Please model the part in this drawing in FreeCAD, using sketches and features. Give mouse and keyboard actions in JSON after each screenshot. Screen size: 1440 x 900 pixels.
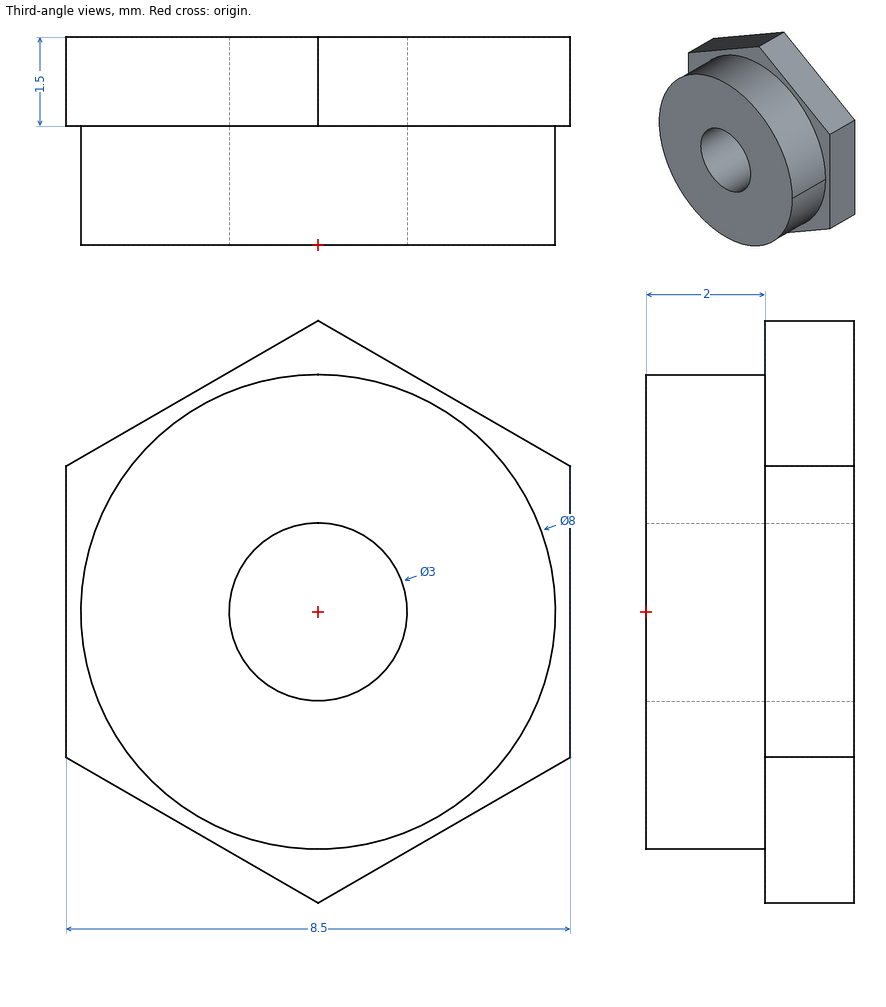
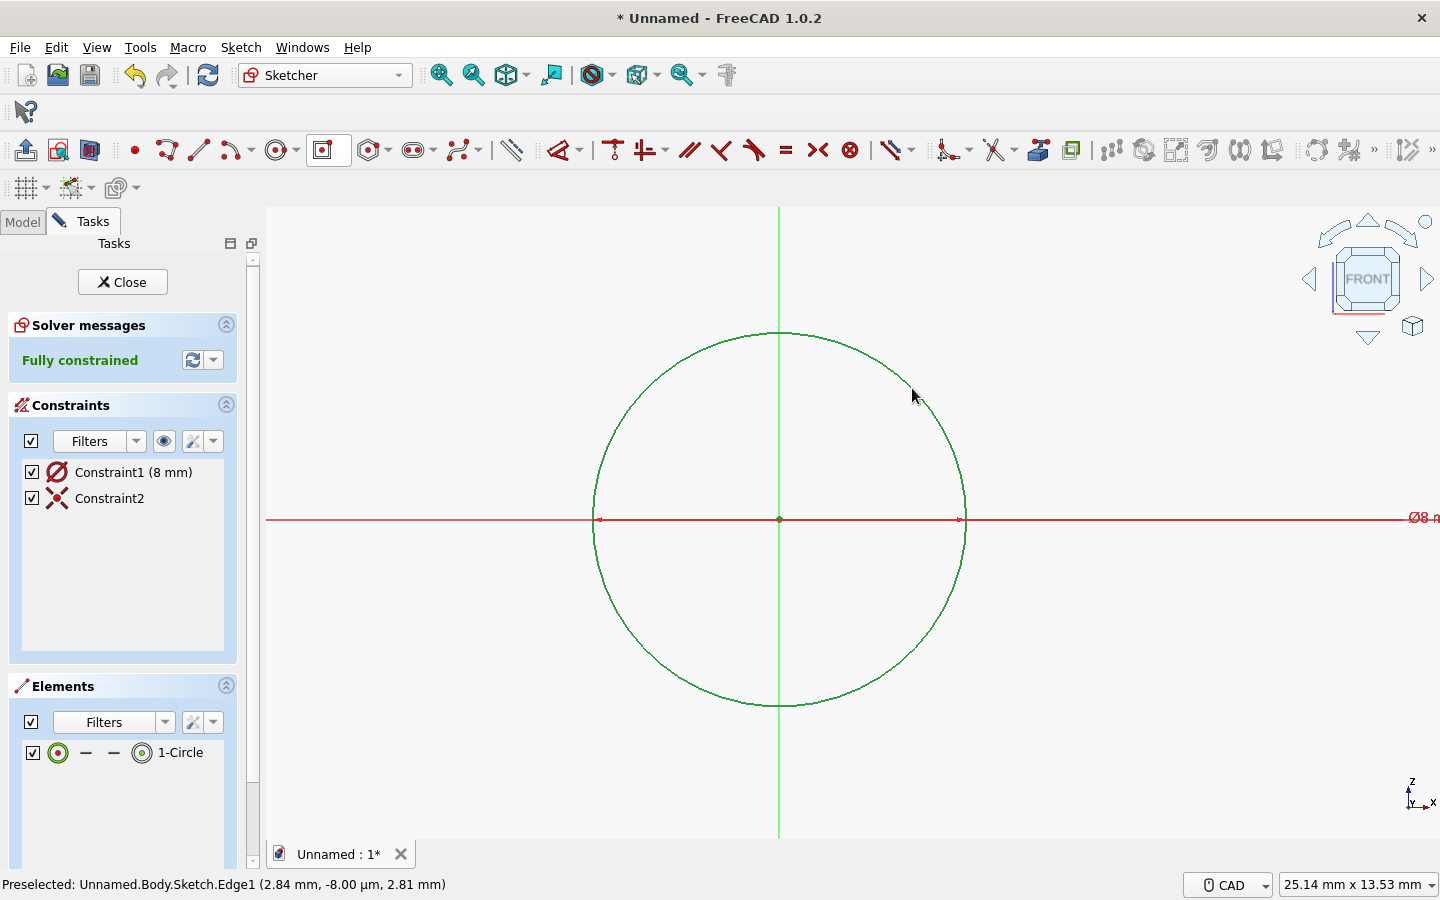
{"action": "left_click", "coordinate": [123, 282]}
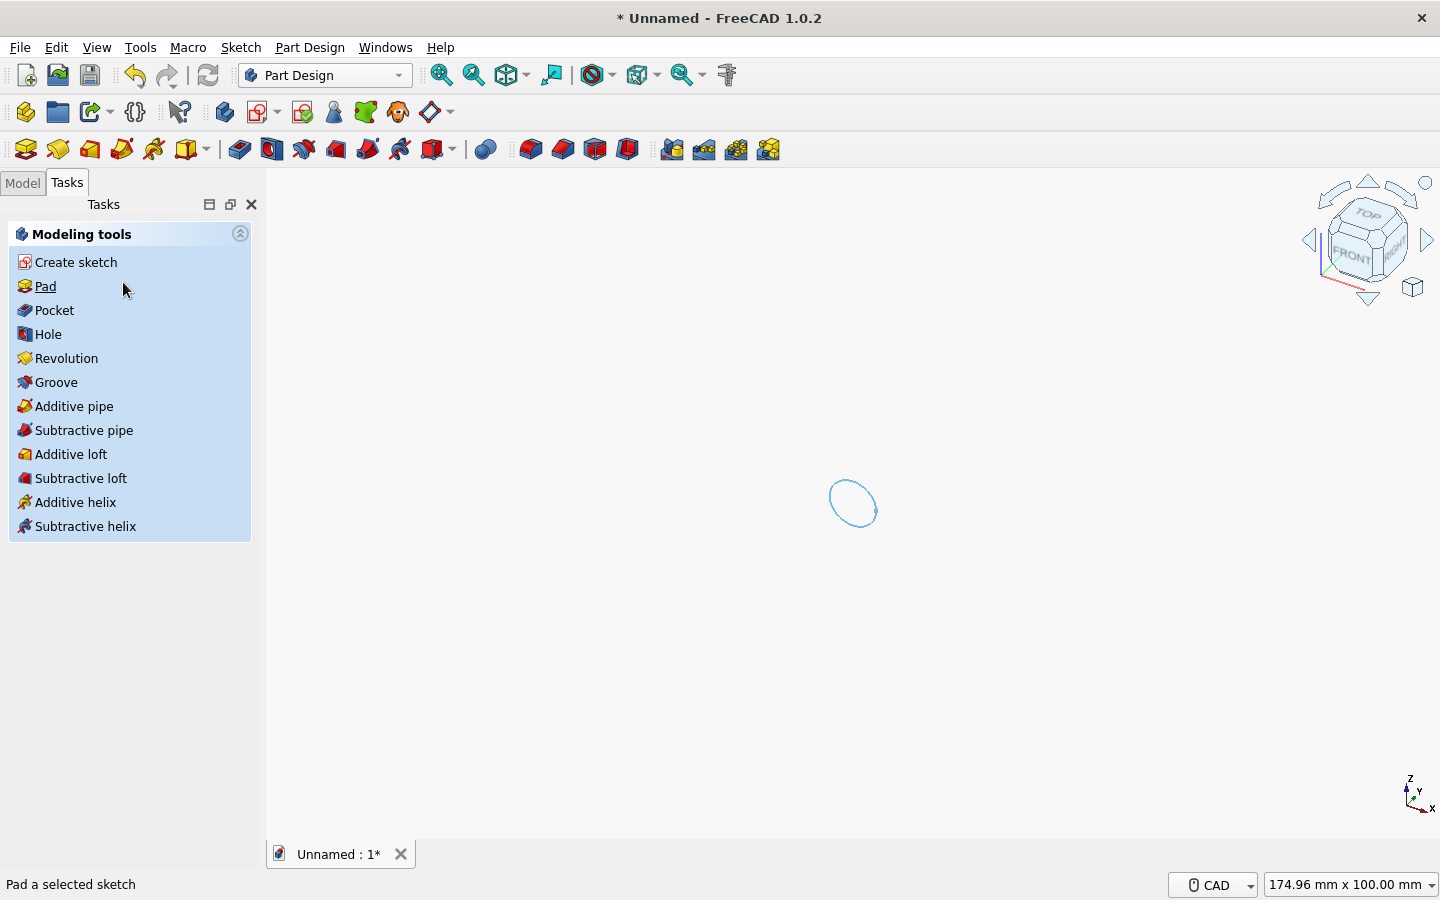
{"action": "left_click", "coordinate": [26, 150]}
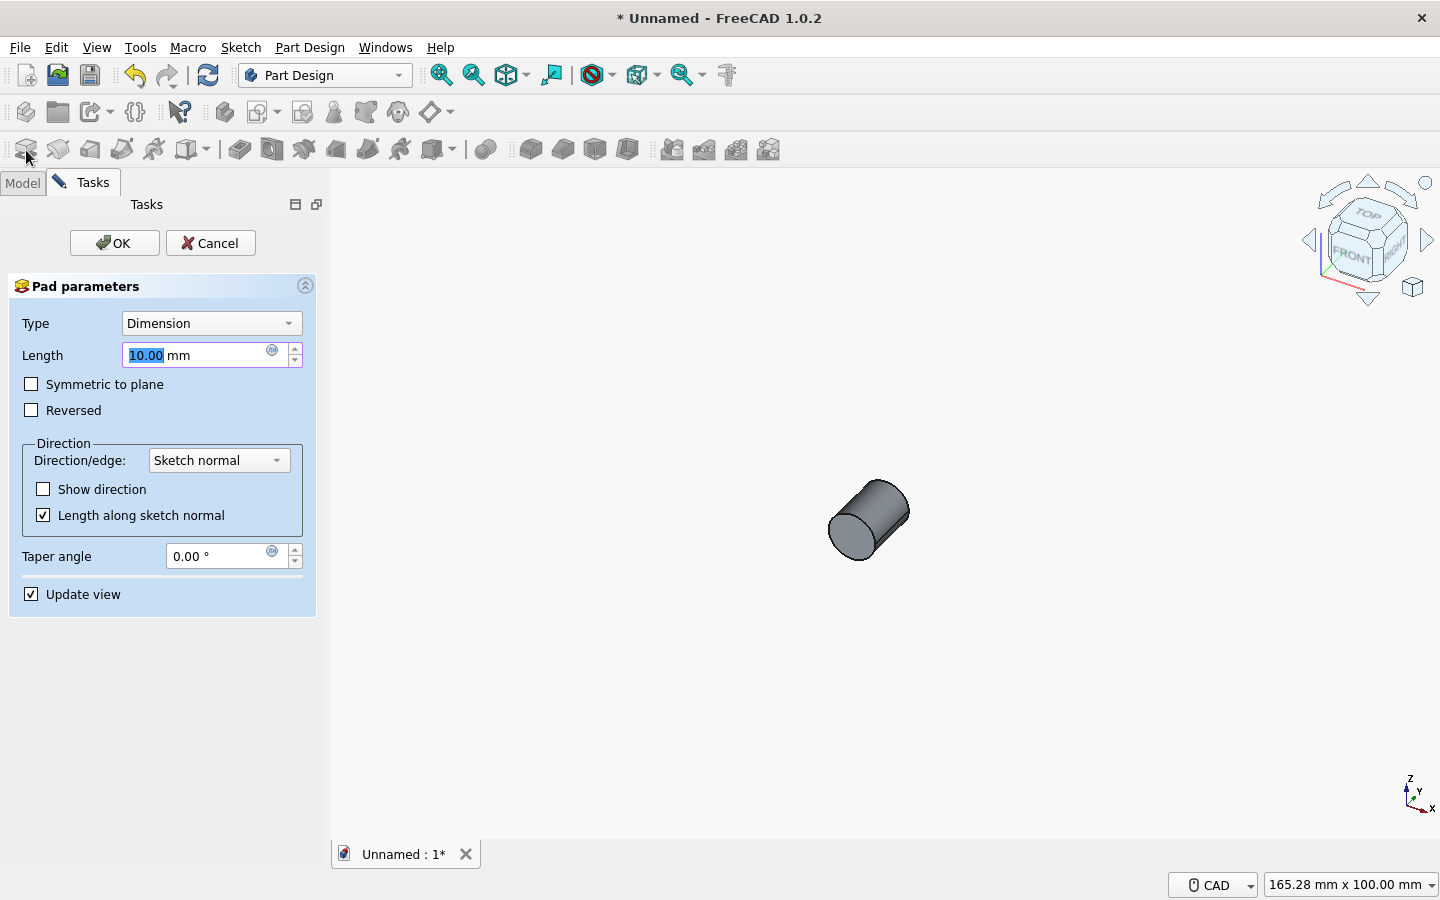
{"action": "type", "text": "2"}
{"action": "key", "text": "Tab"}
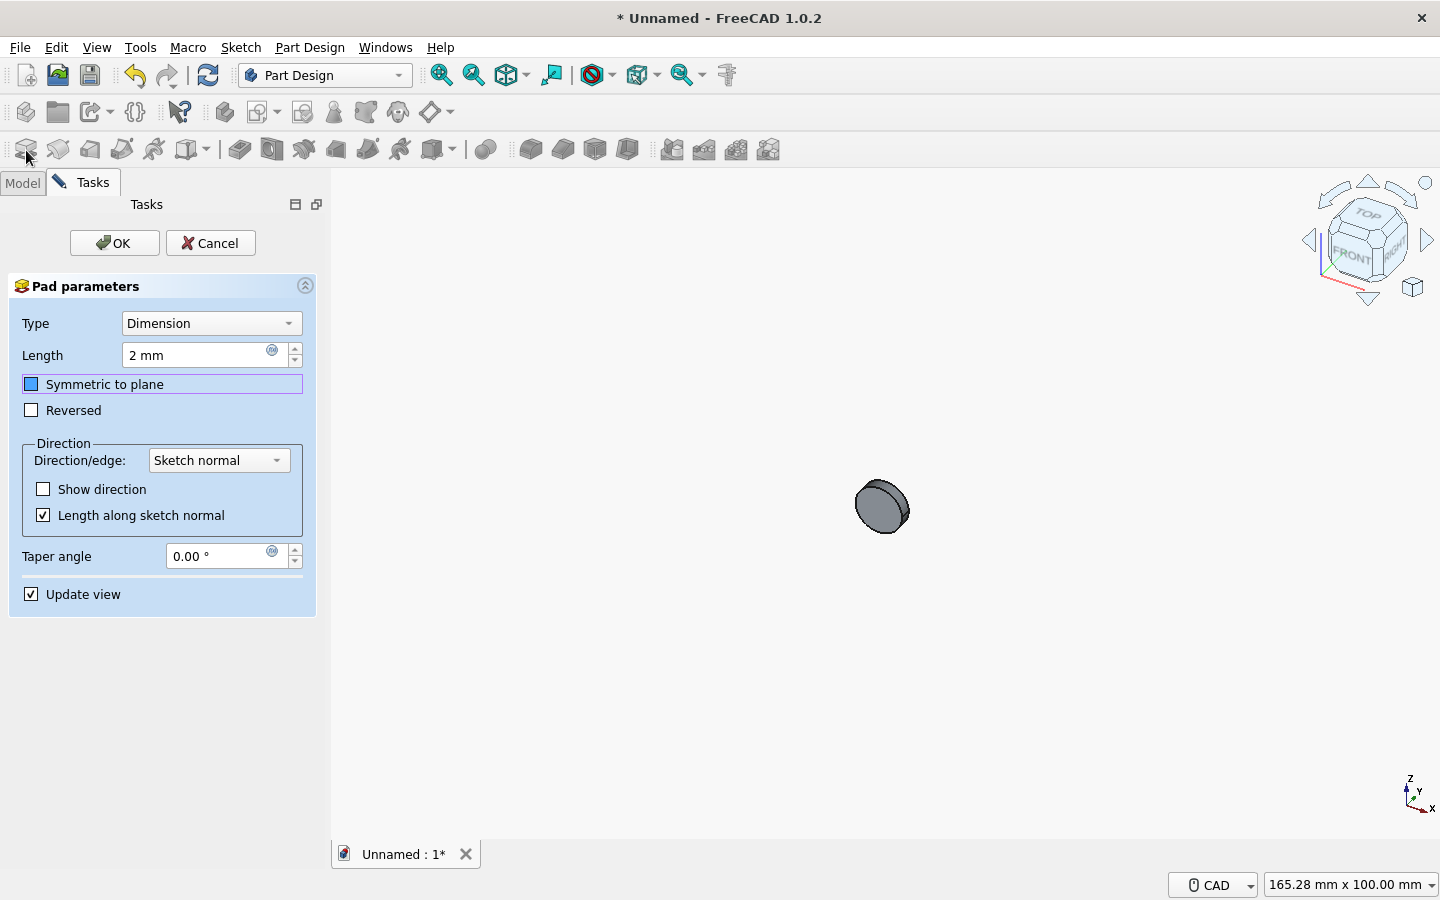
{"action": "left_click", "coordinate": [30, 410]}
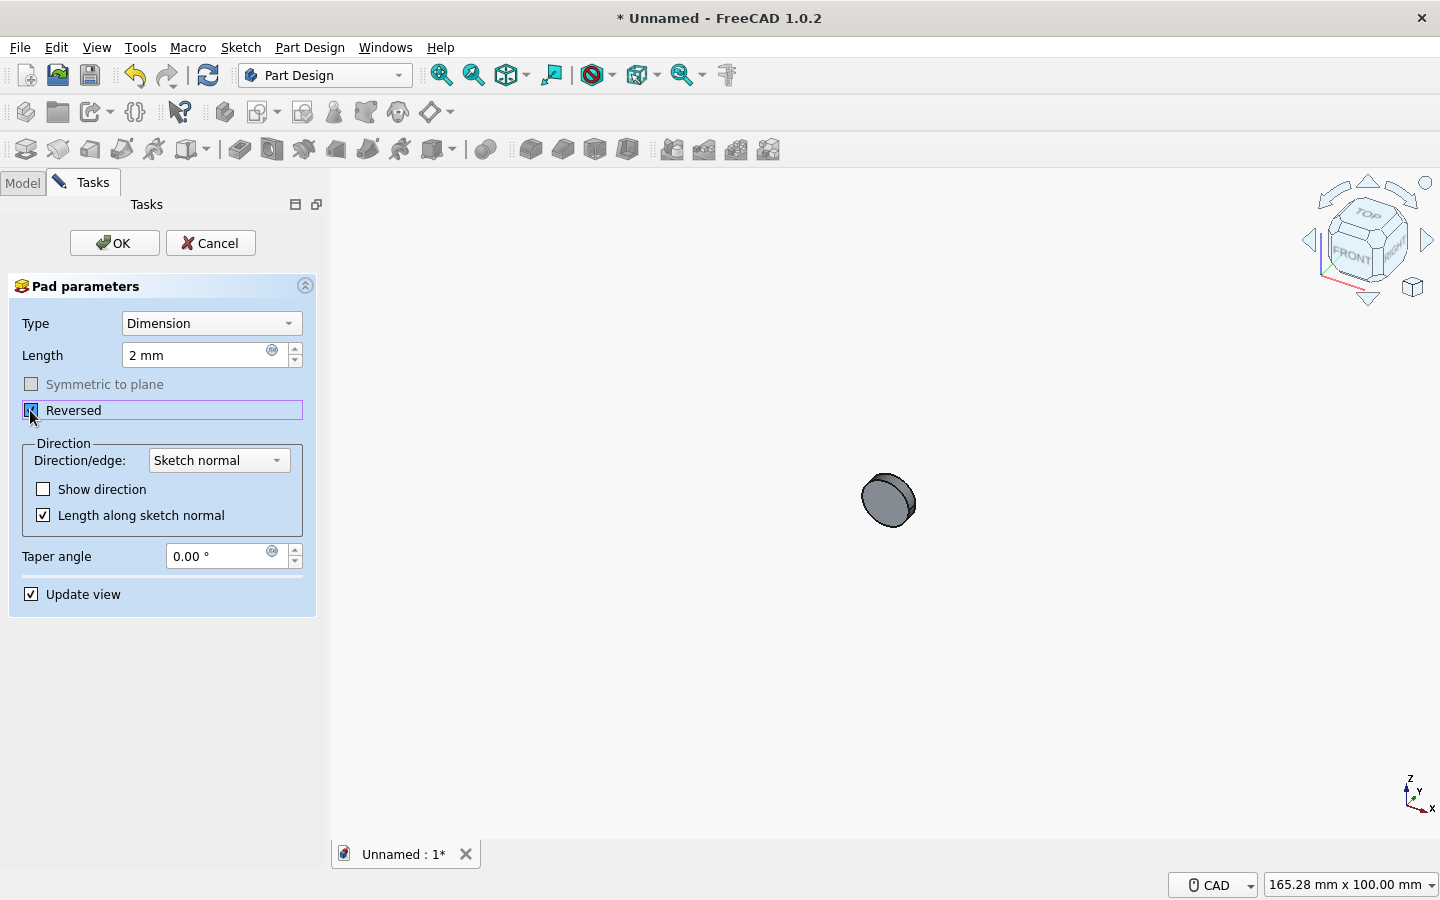
{"action": "left_click", "coordinate": [115, 243]}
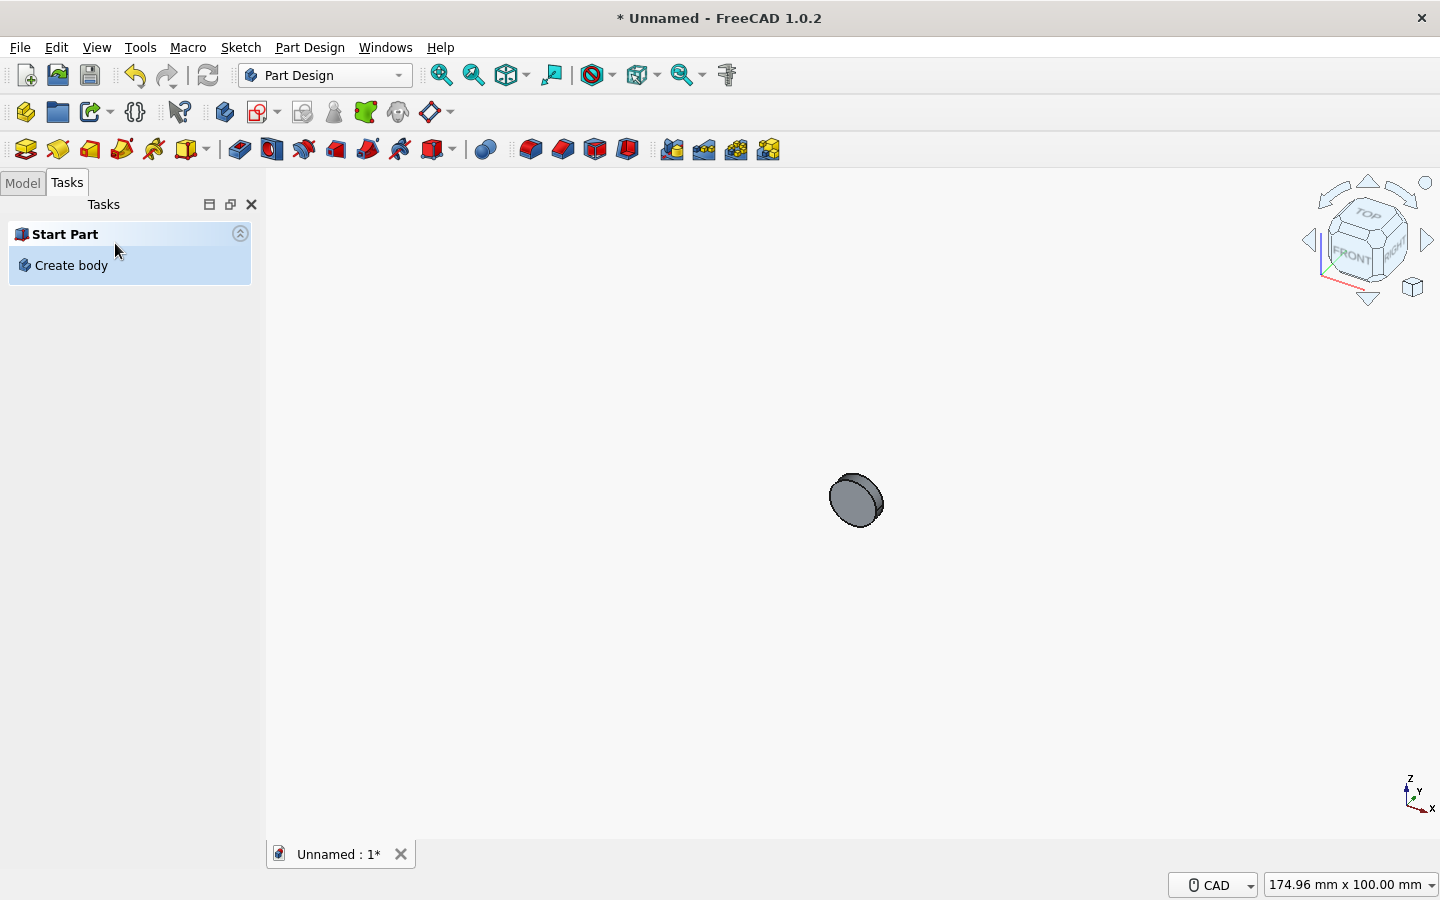
{"action": "left_click", "coordinate": [442, 76]}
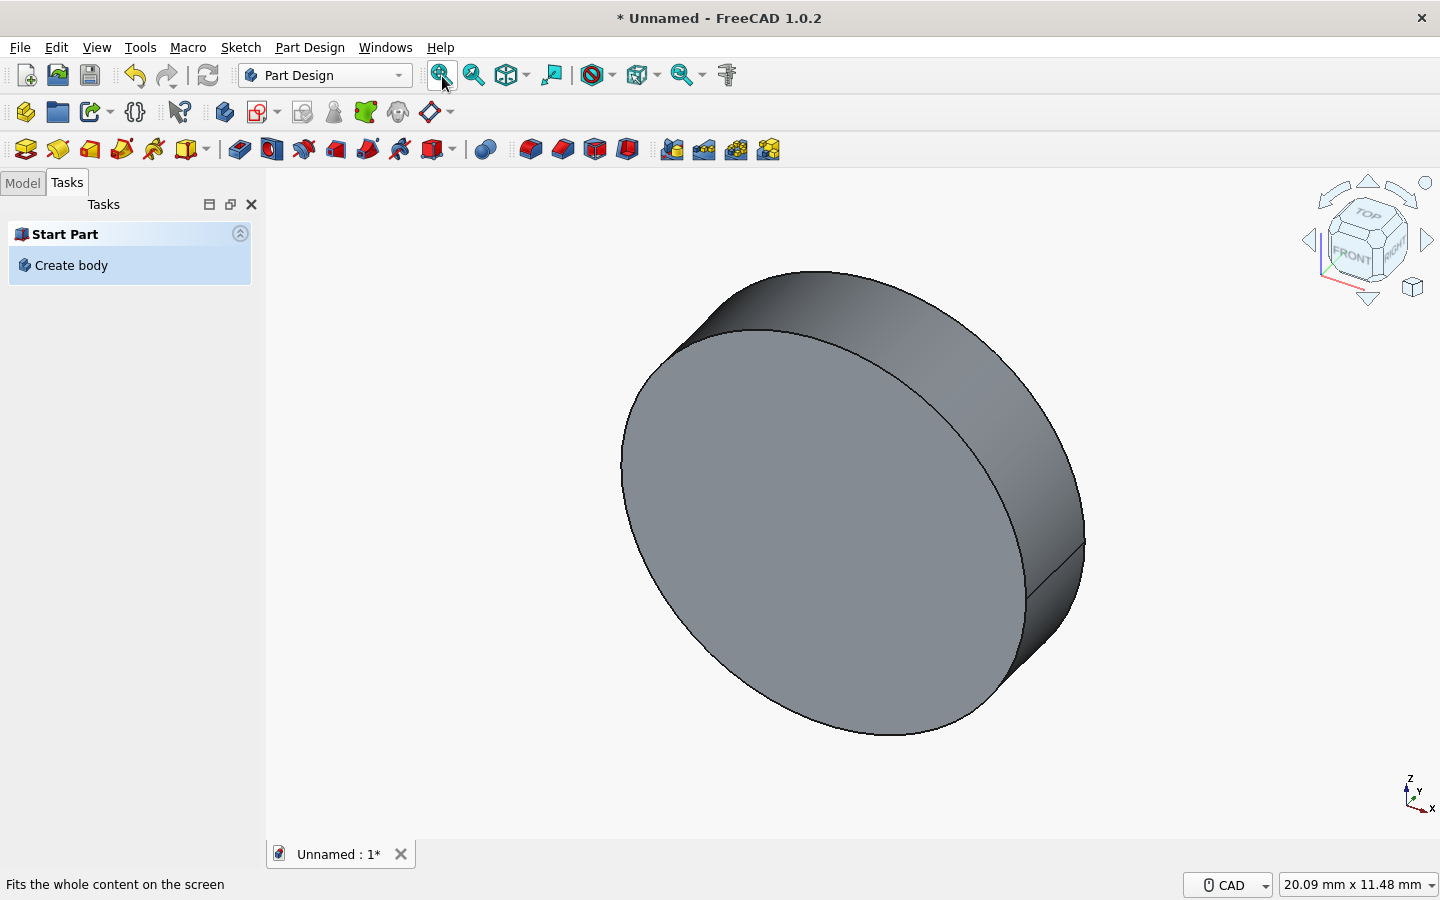
{"action": "key", "text": "4"}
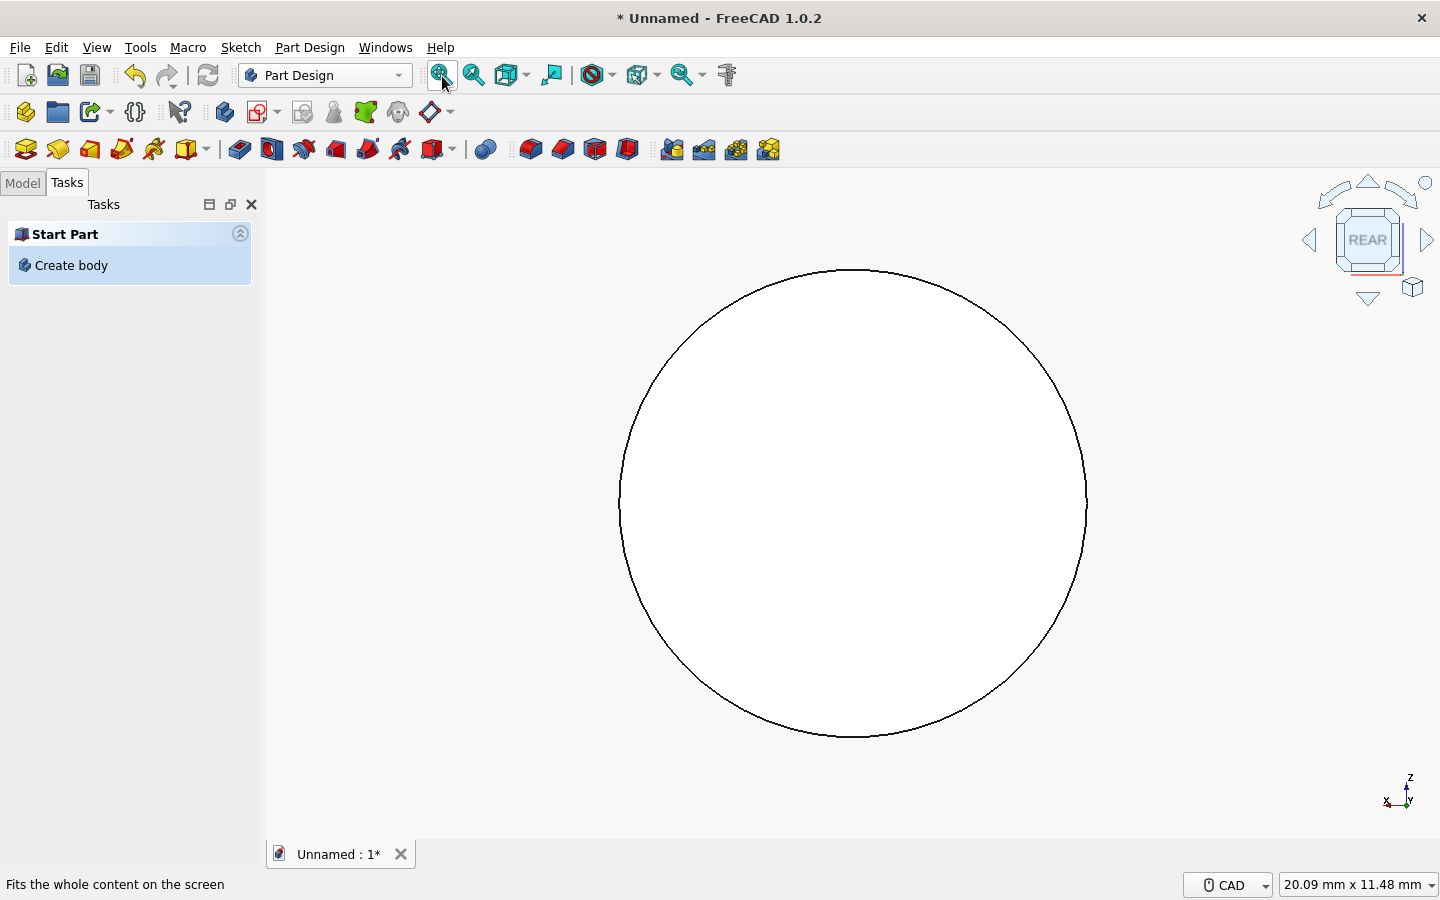
{"action": "left_click", "coordinate": [853, 503]}